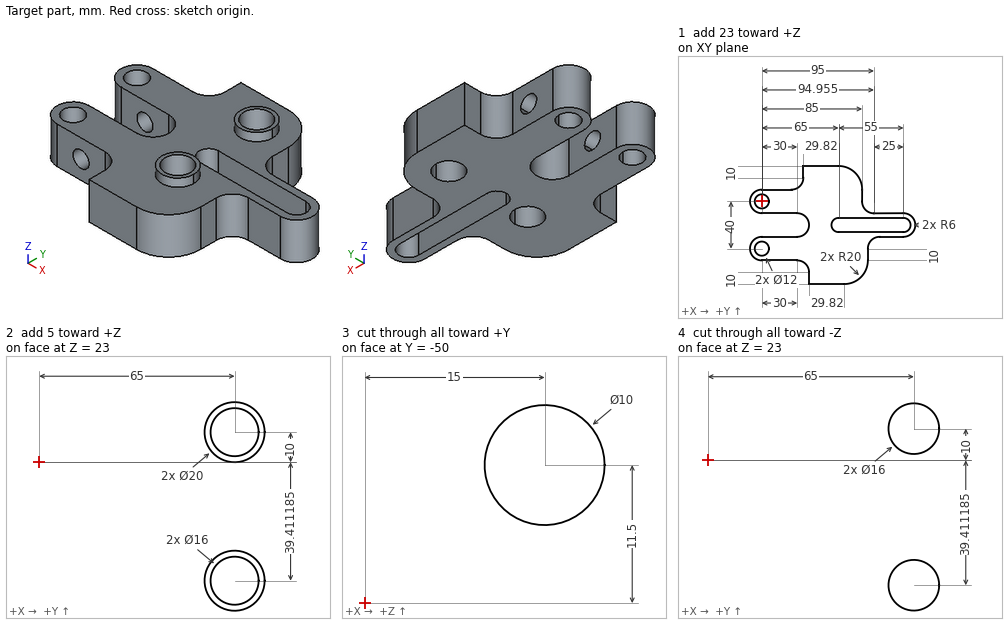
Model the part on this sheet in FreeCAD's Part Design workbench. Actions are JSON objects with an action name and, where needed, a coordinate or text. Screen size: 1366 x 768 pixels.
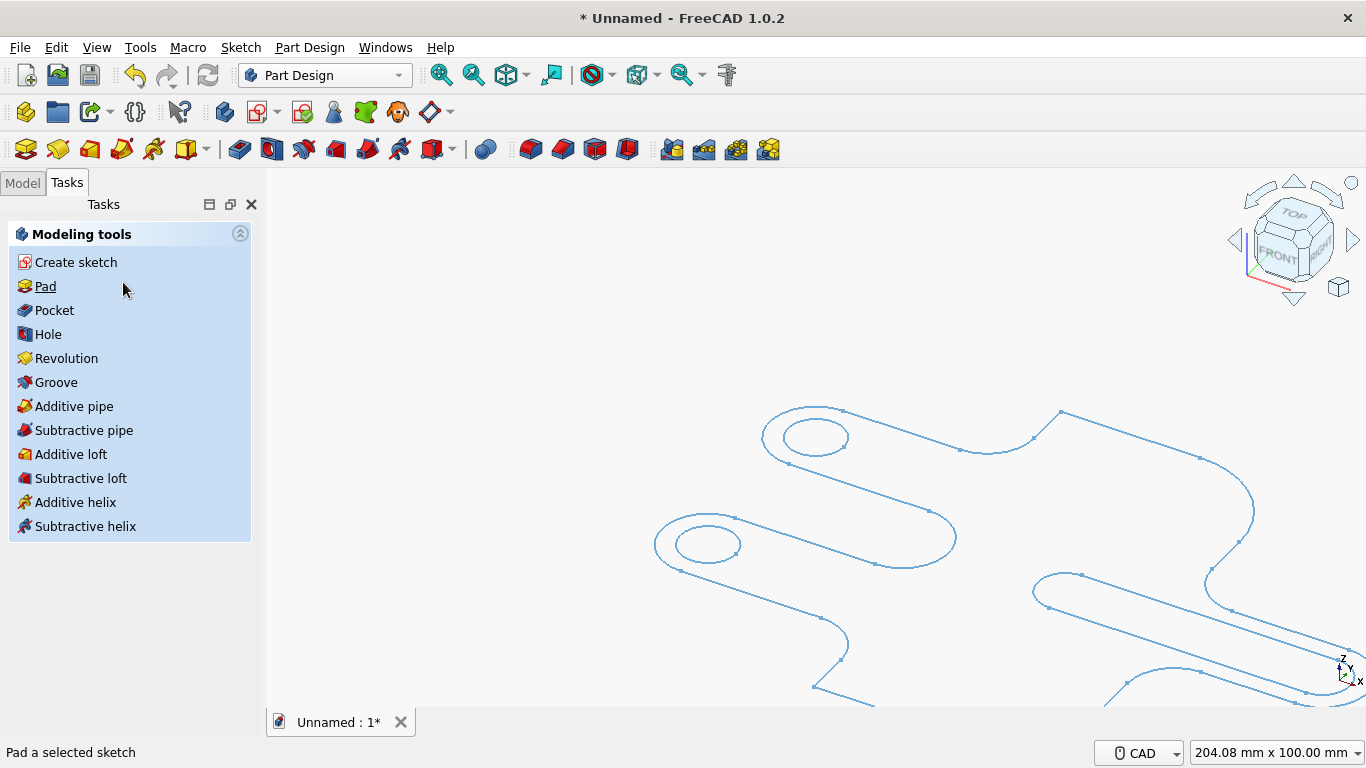
{"action": "left_click", "coordinate": [26, 150]}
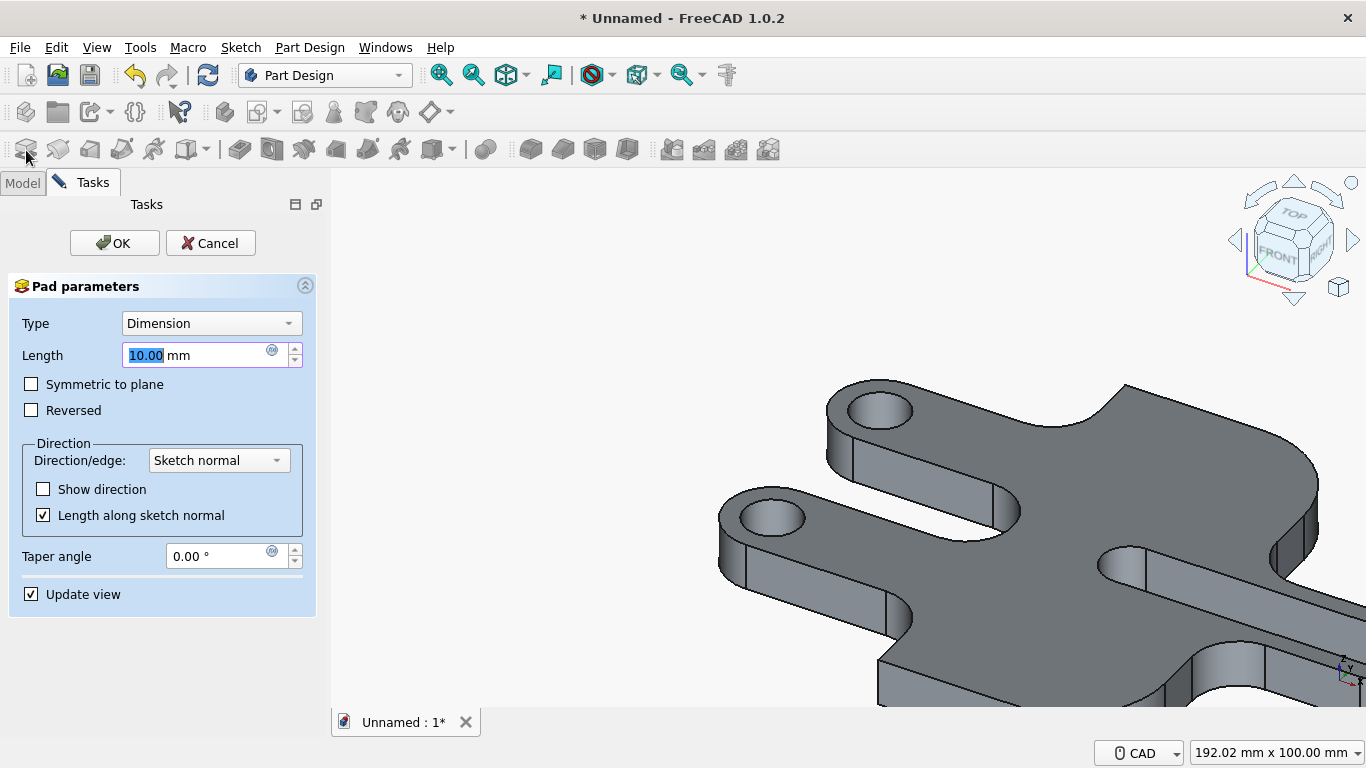
{"action": "type", "text": "23"}
{"action": "key", "text": "Tab"}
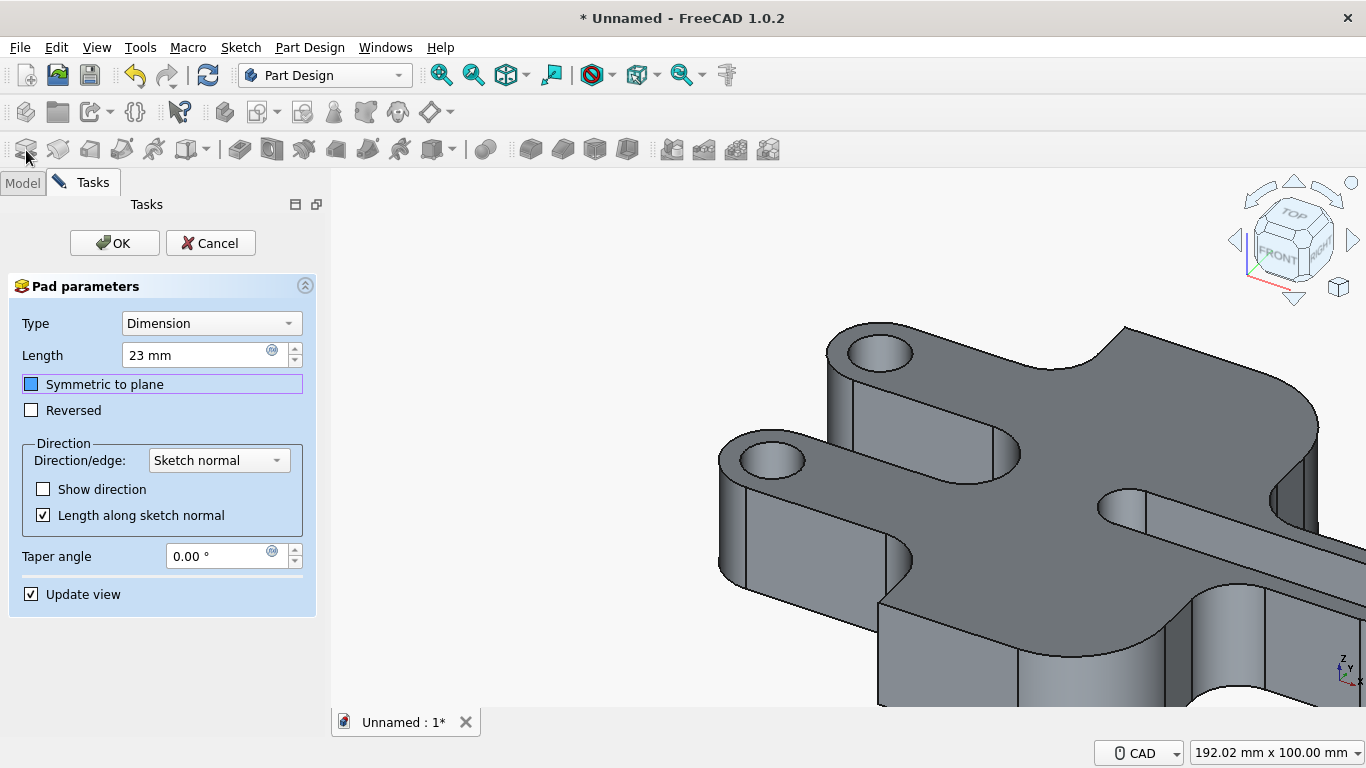
{"action": "left_click", "coordinate": [115, 243]}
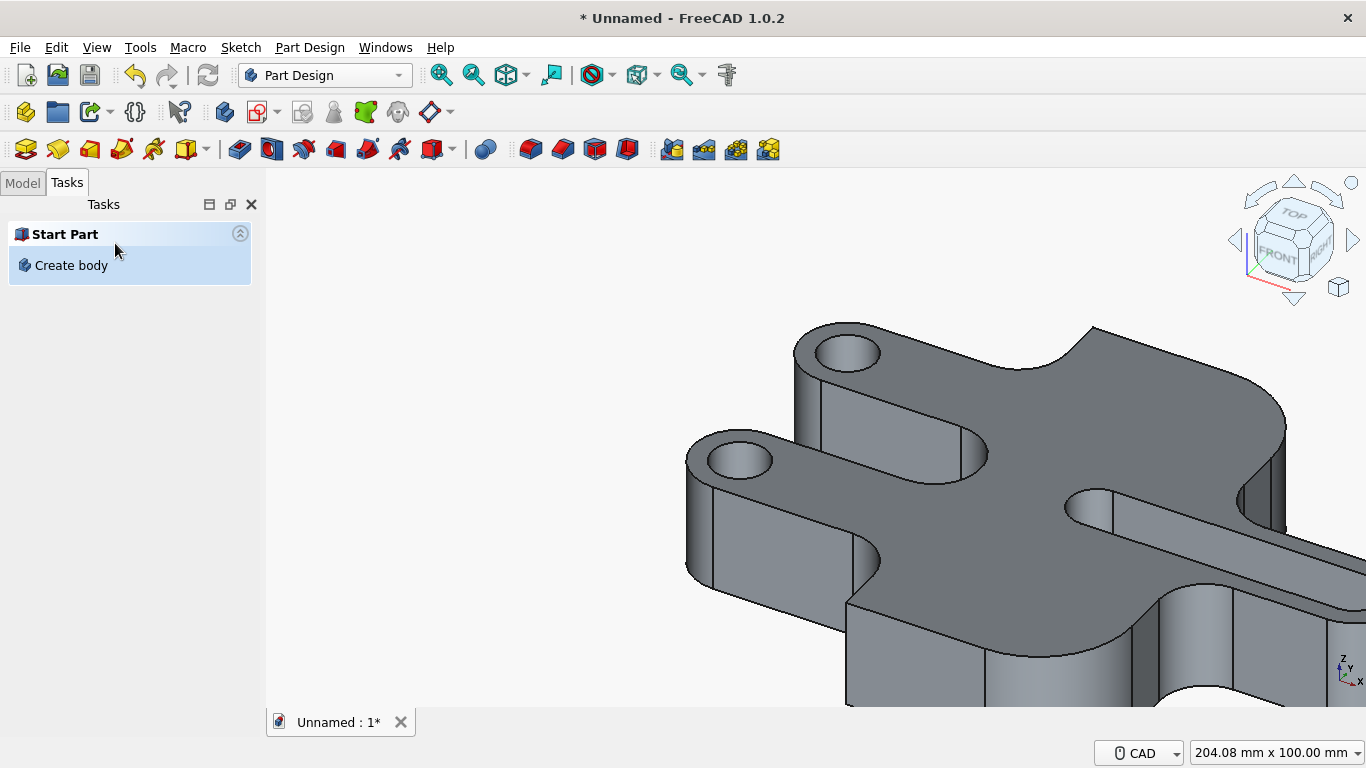
{"action": "left_click", "coordinate": [442, 76]}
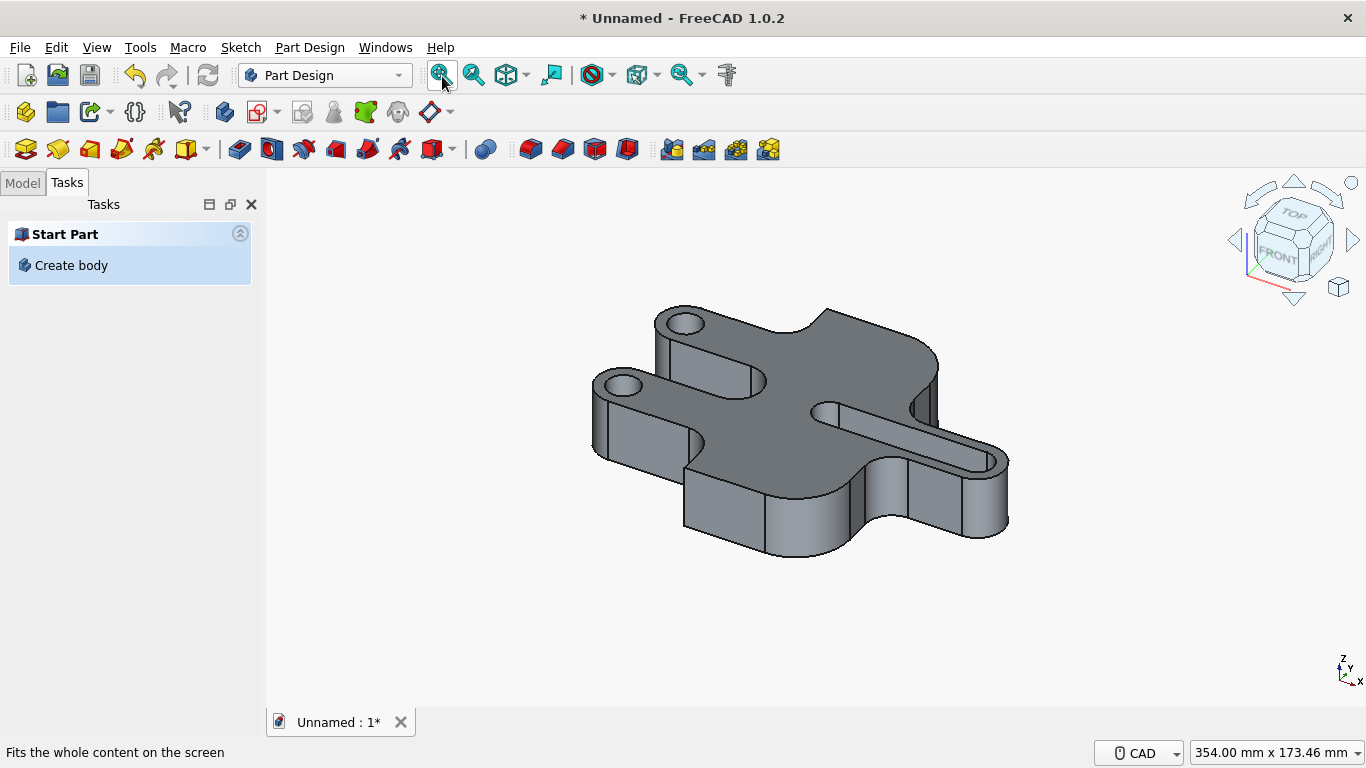
{"action": "left_click", "coordinate": [860, 363]}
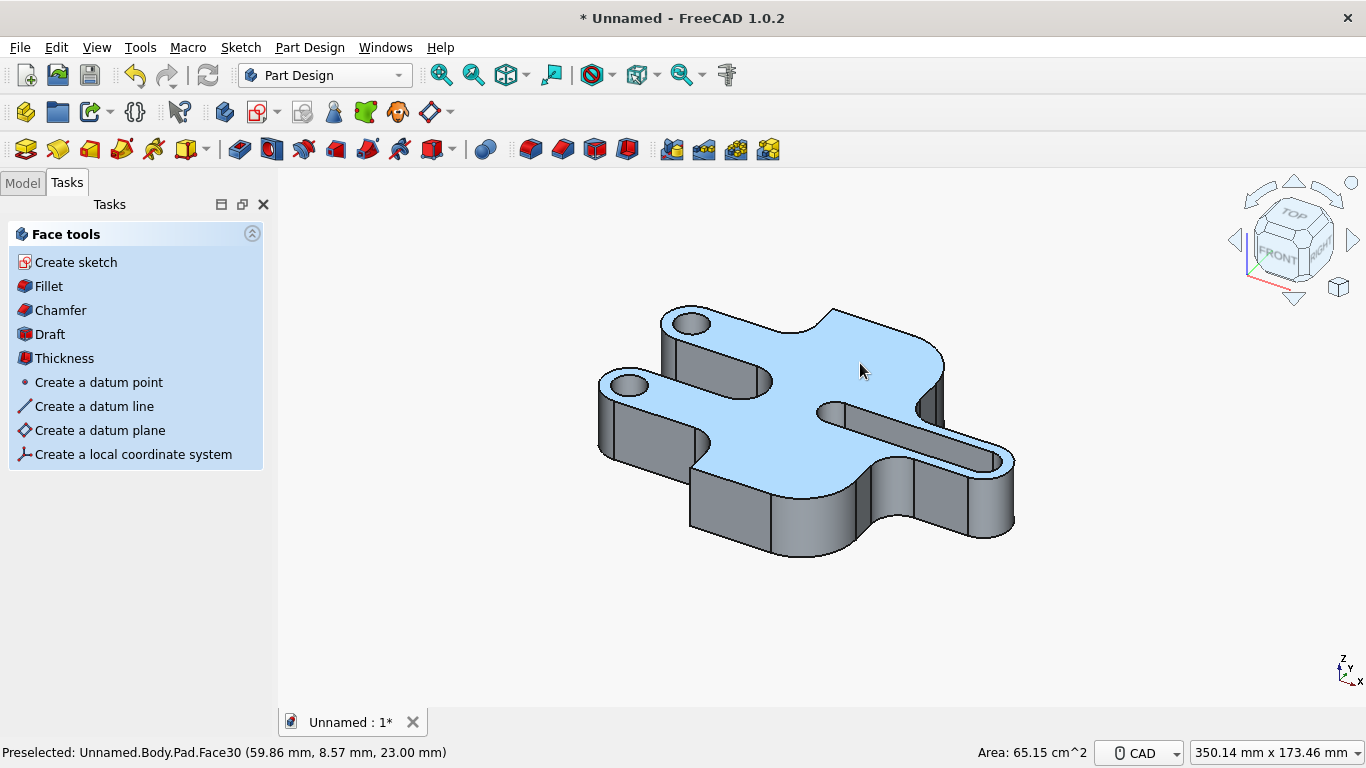
{"action": "left_click", "coordinate": [258, 112]}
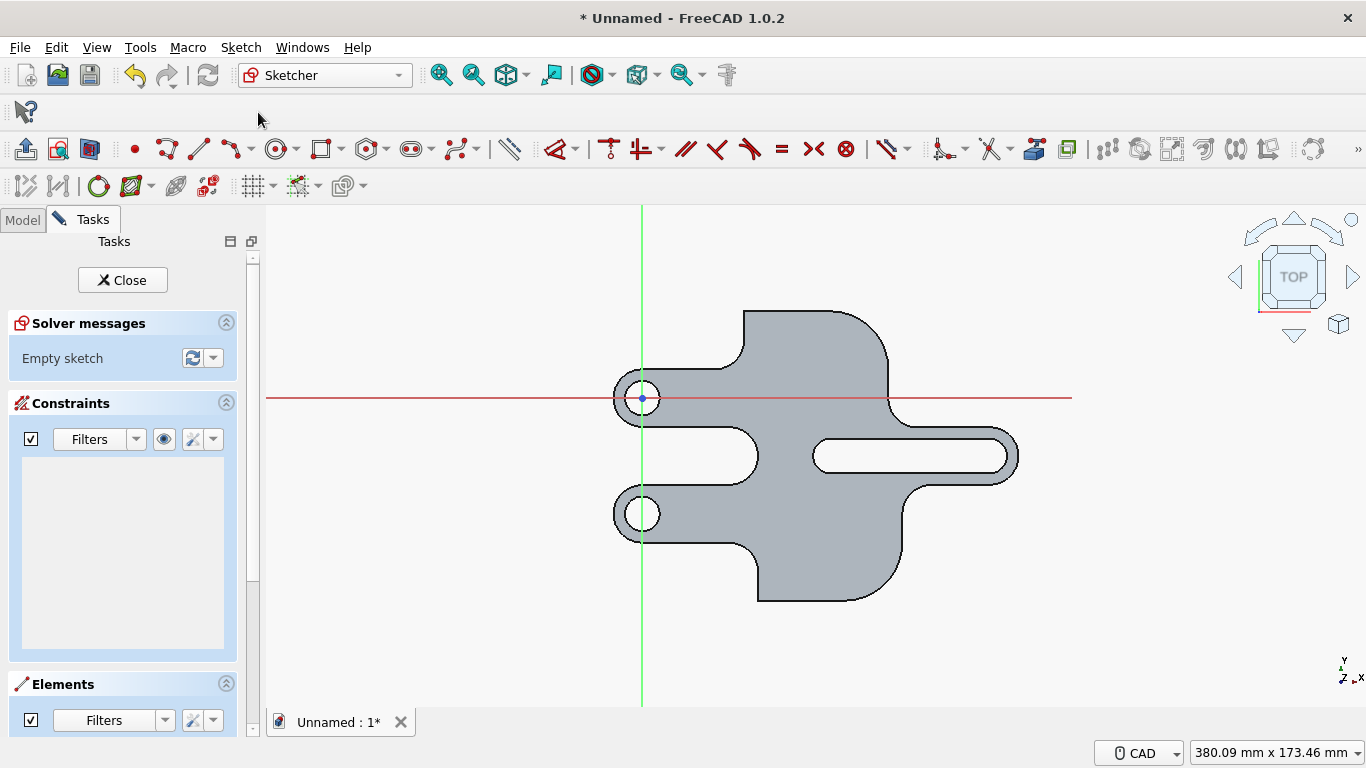
{"action": "scroll", "coordinate": [758, 410], "scroll_direction": "up", "scroll_amount": 2}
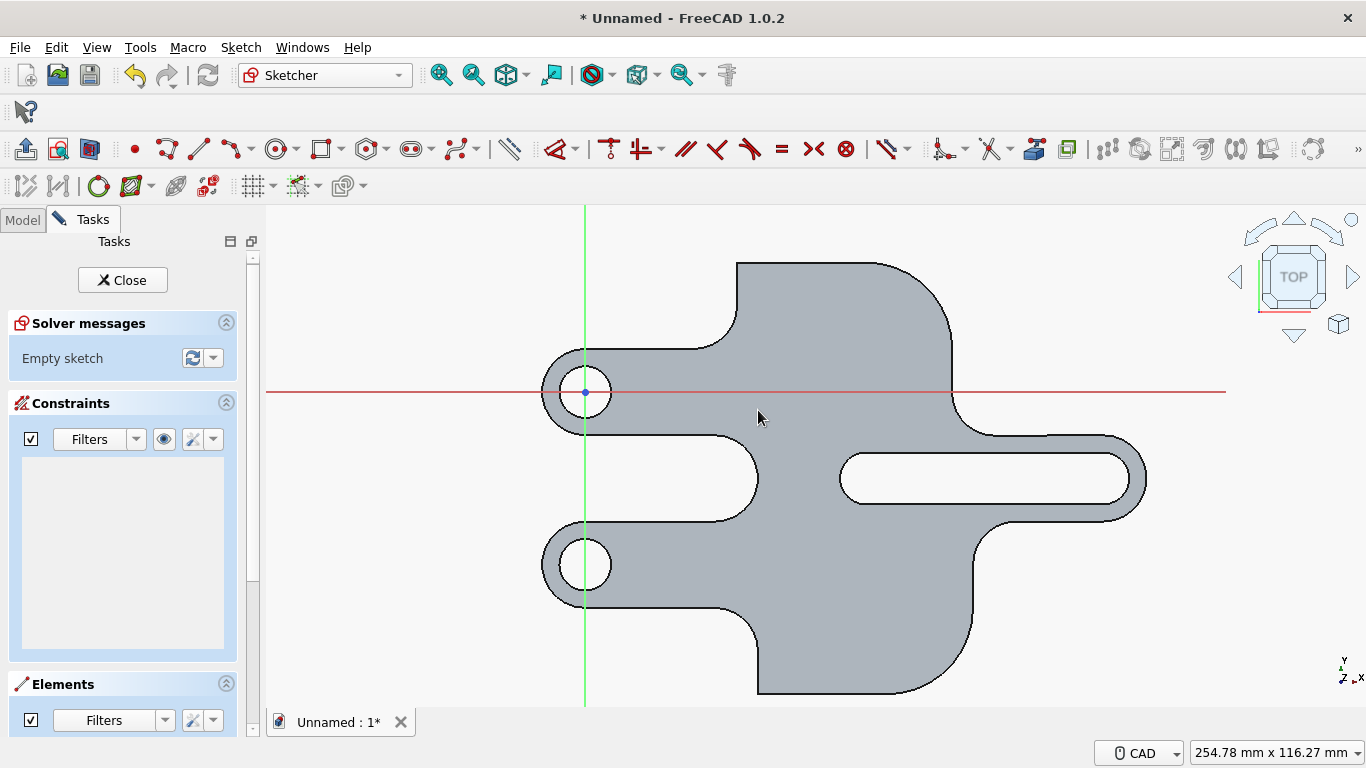
{"action": "left_click", "coordinate": [276, 150]}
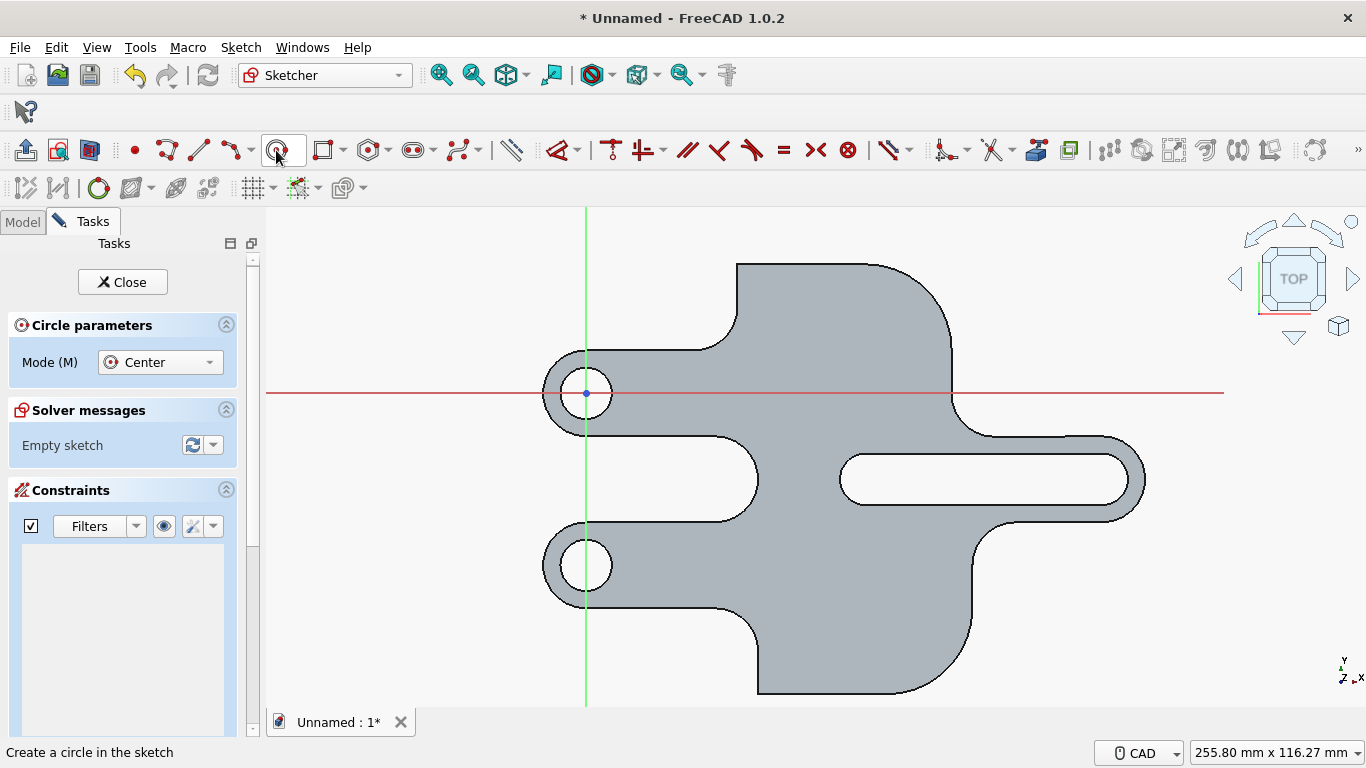
{"action": "left_click", "coordinate": [866, 350]}
{"action": "mouse_move", "coordinate": [896, 320]}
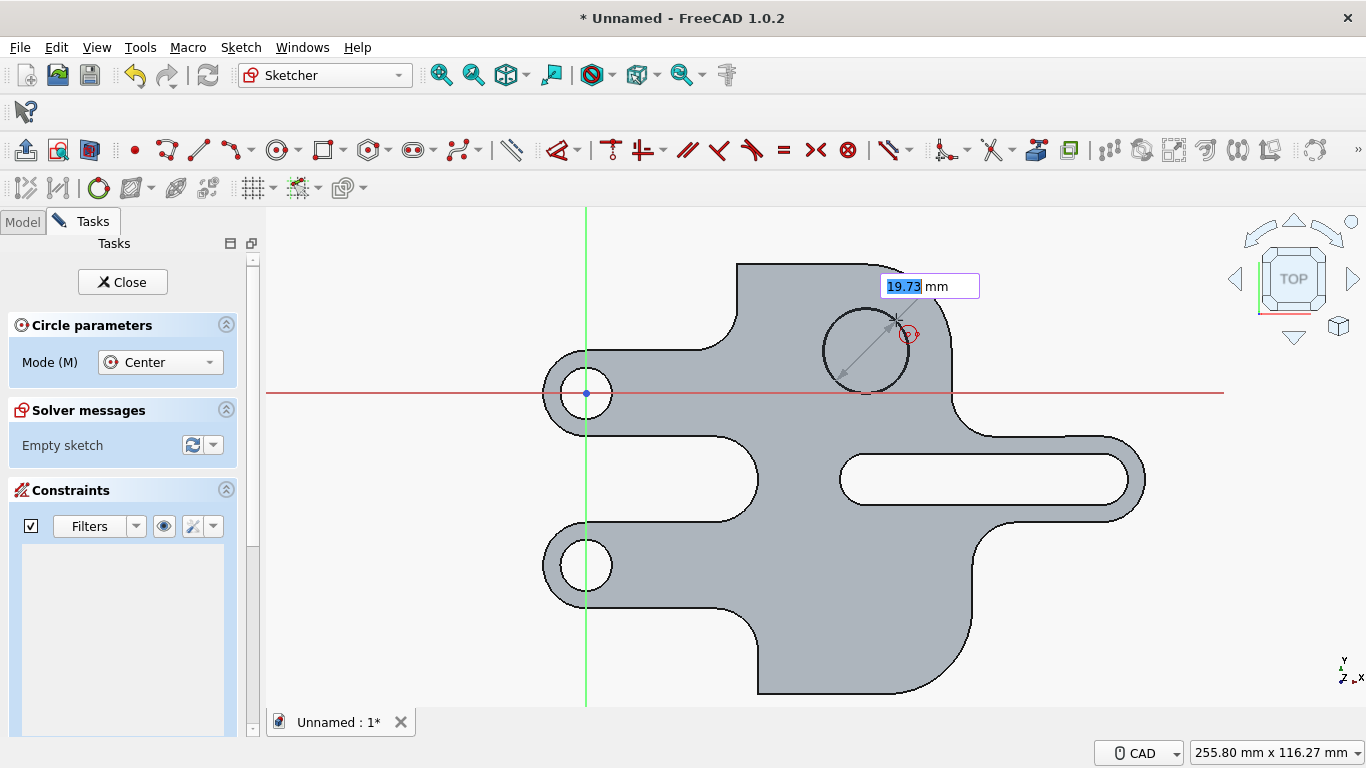
{"action": "type", "text": "20"}
{"action": "key", "text": "Return"}